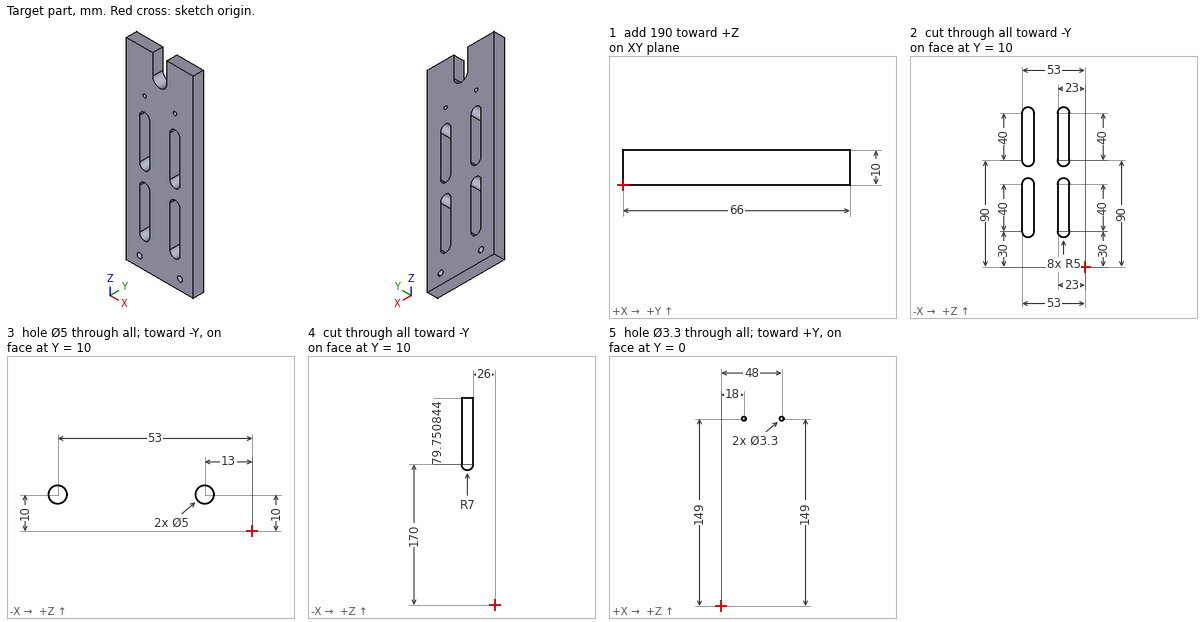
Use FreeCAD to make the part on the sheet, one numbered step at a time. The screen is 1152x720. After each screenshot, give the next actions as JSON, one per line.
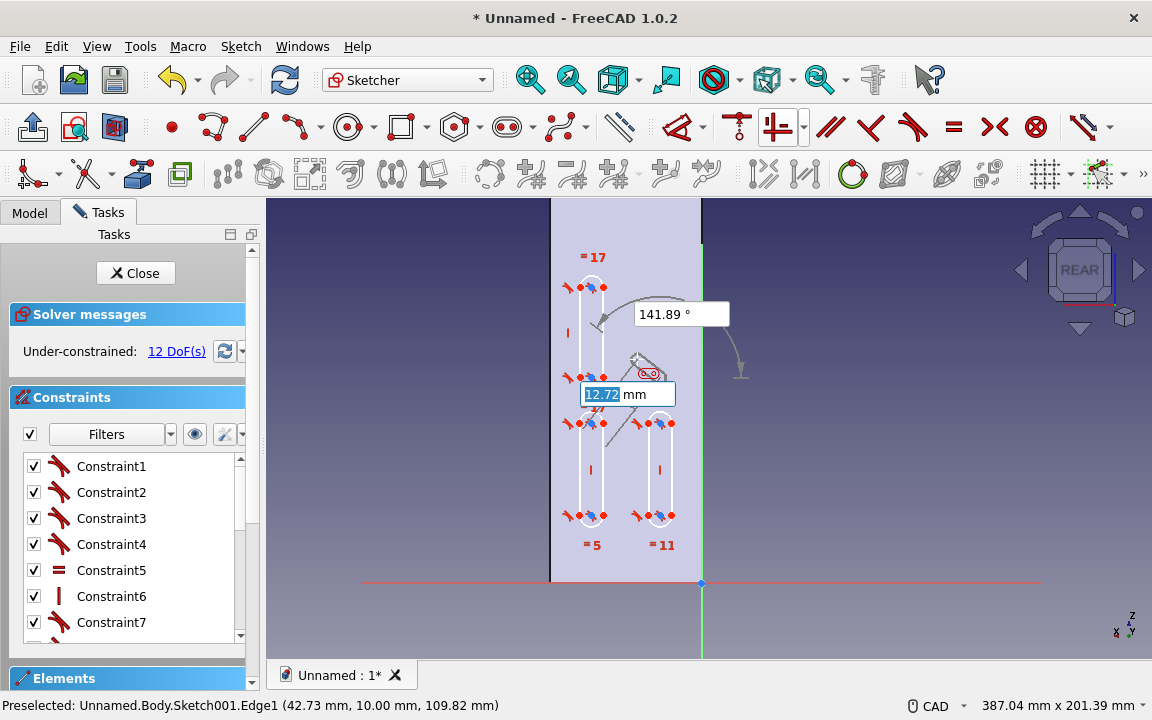
{"action": "left_click", "coordinate": [660, 286]}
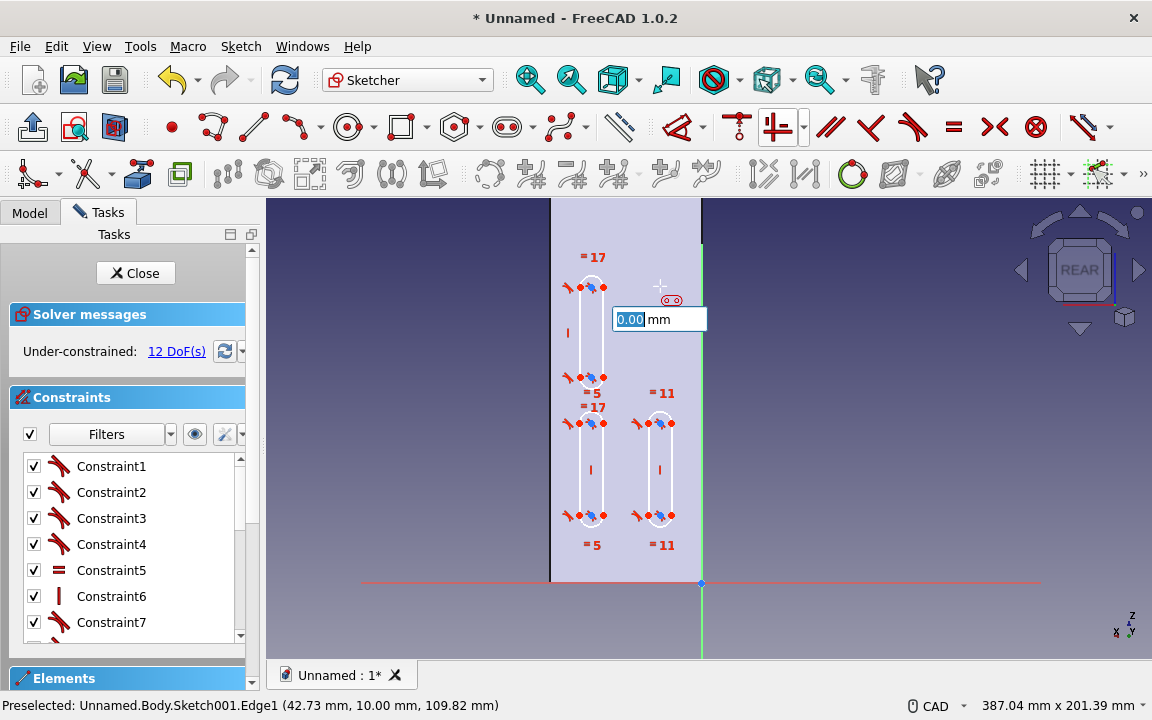
{"action": "scroll", "coordinate": [672, 332], "scroll_direction": "up", "scroll_amount": 2}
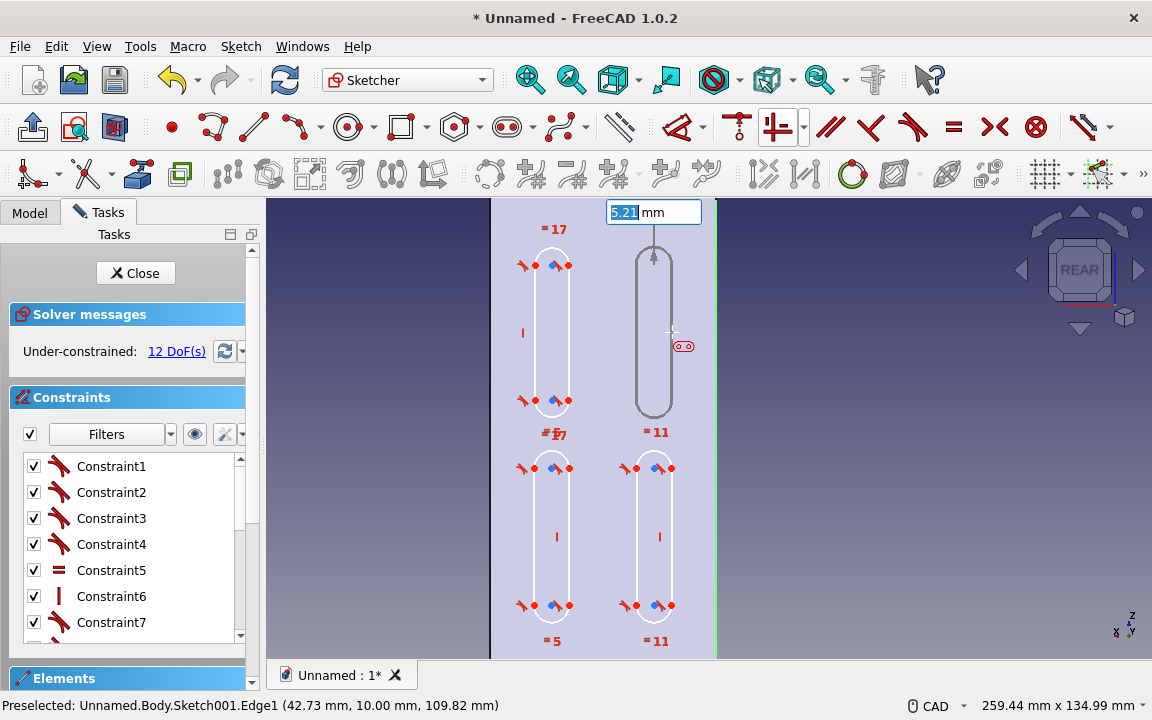
{"action": "left_click", "coordinate": [671, 331]}
{"action": "key", "text": "Escape"}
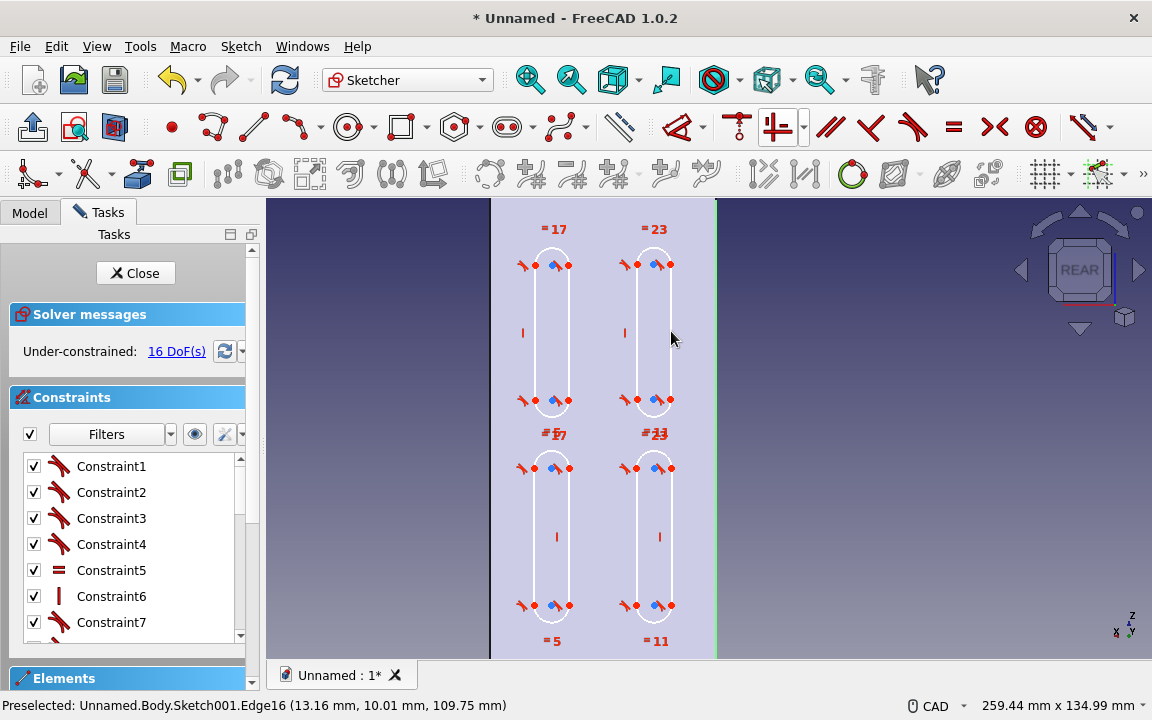
{"action": "left_click", "coordinate": [541, 619]}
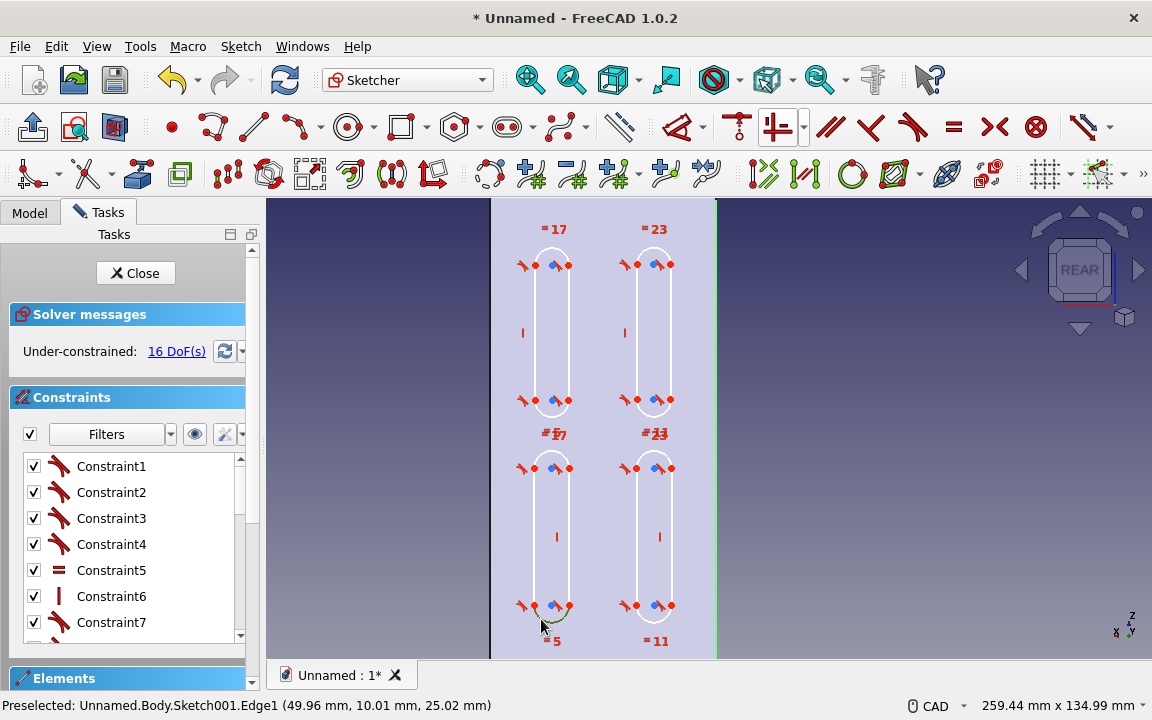
{"action": "left_click", "coordinate": [644, 619]}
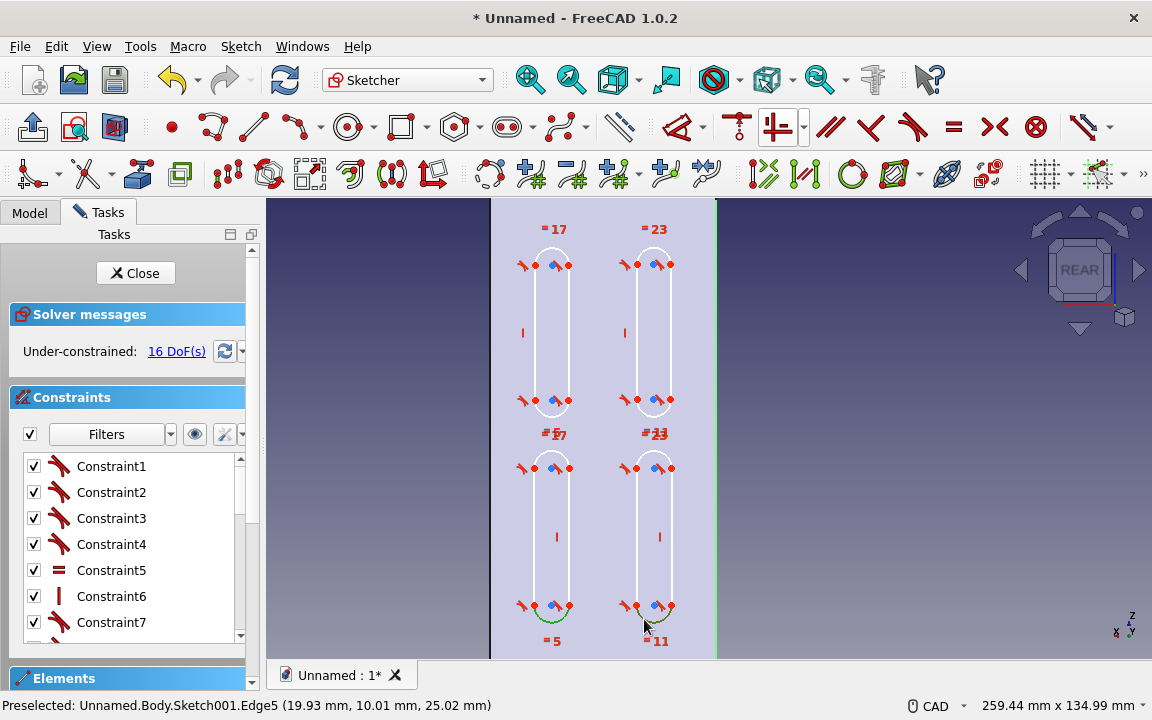
{"action": "left_click", "coordinate": [542, 414]}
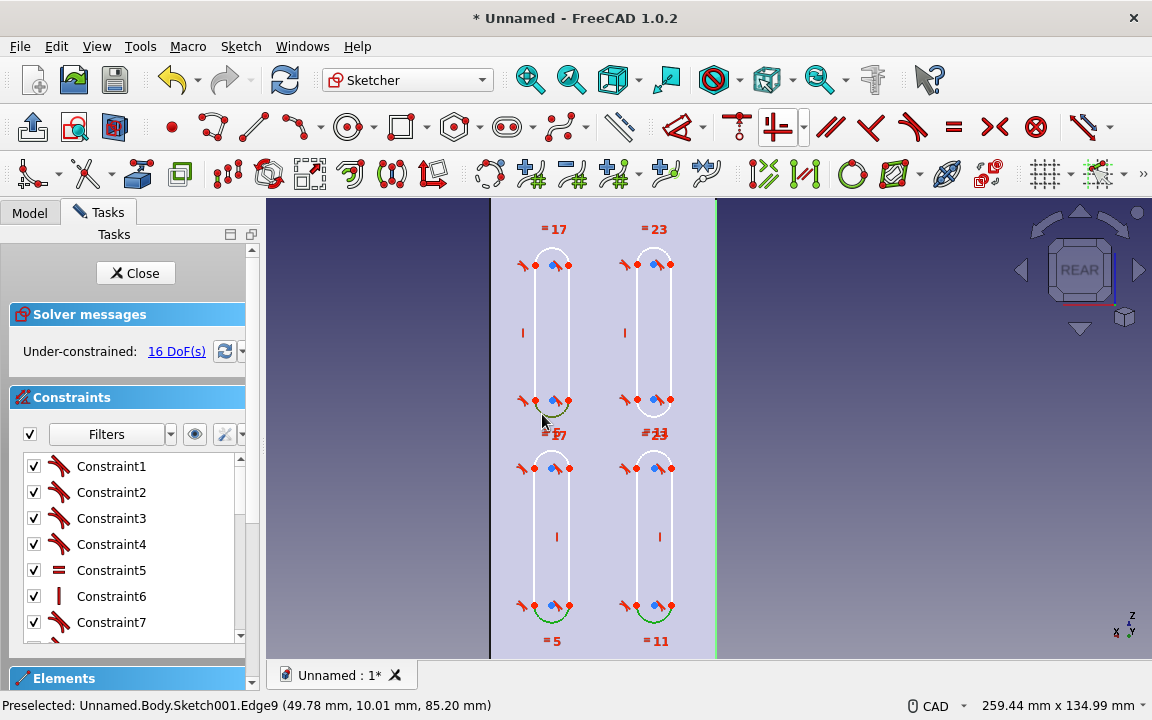
{"action": "left_click", "coordinate": [644, 414]}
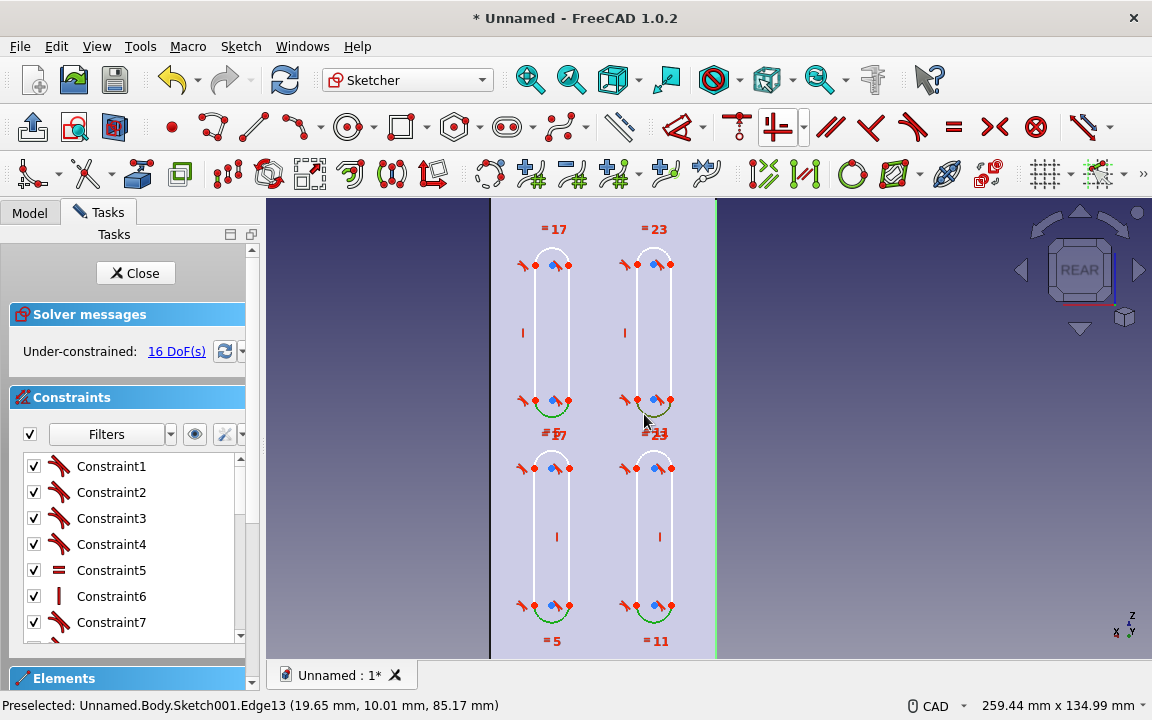
{"action": "left_click", "coordinate": [954, 128]}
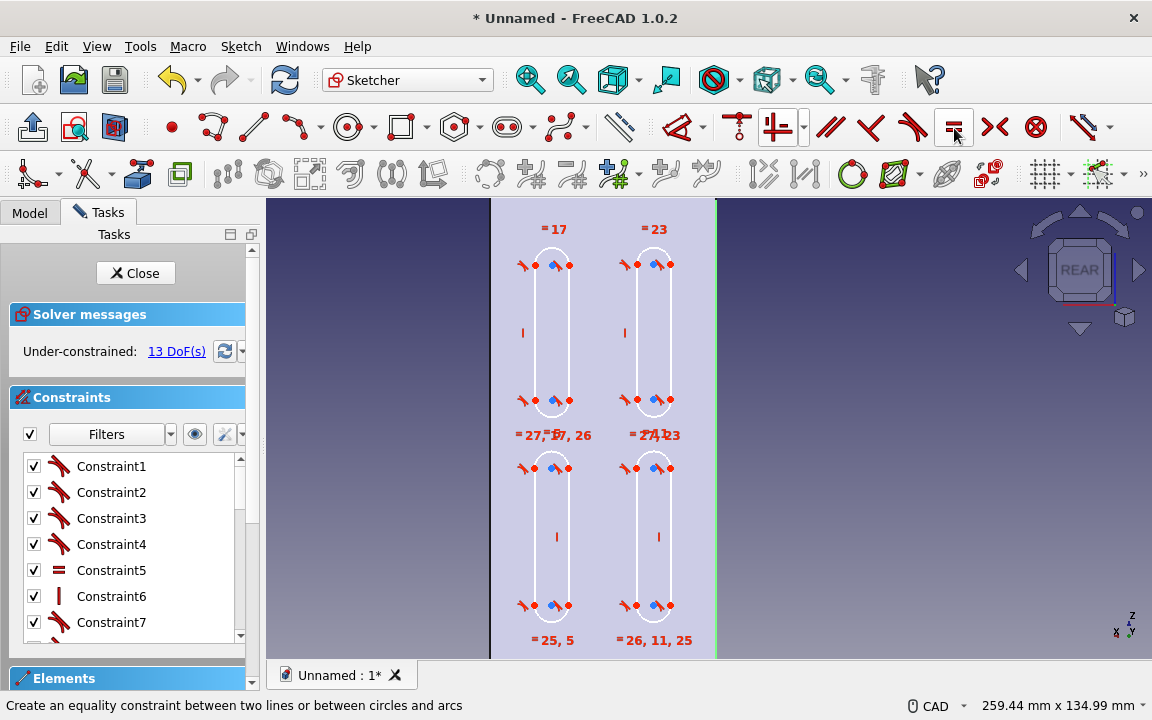
{"action": "left_click", "coordinate": [676, 128]}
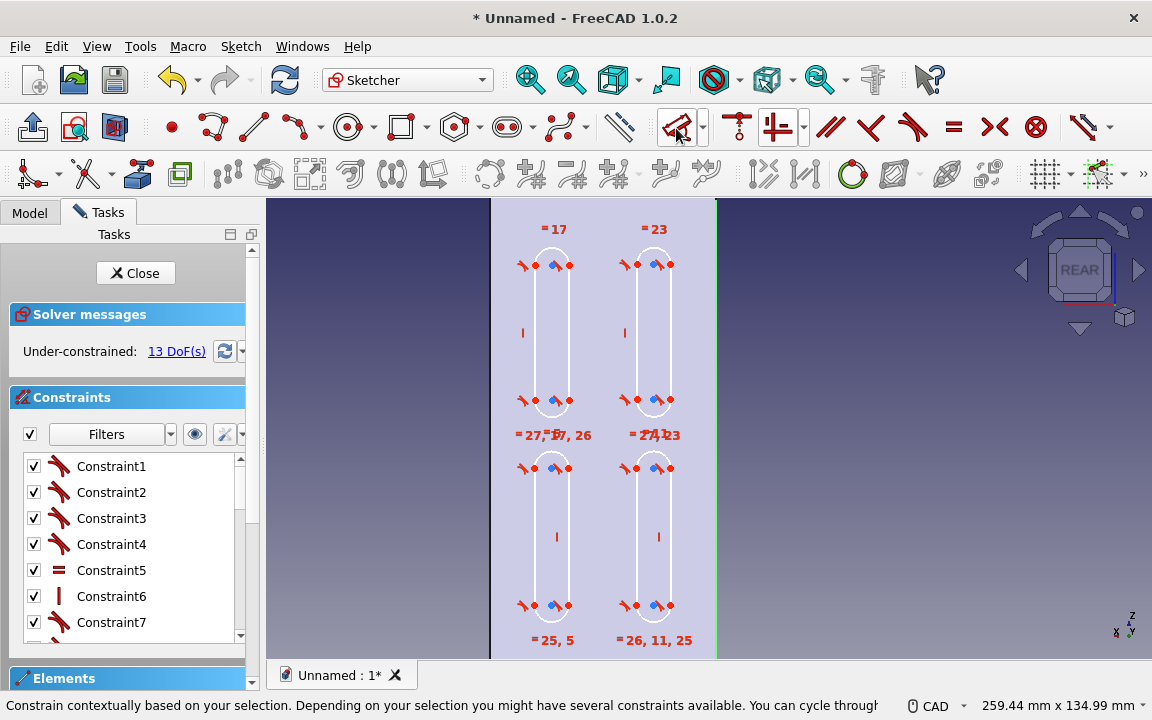
{"action": "scroll", "coordinate": [542, 619], "scroll_direction": "up", "scroll_amount": 5}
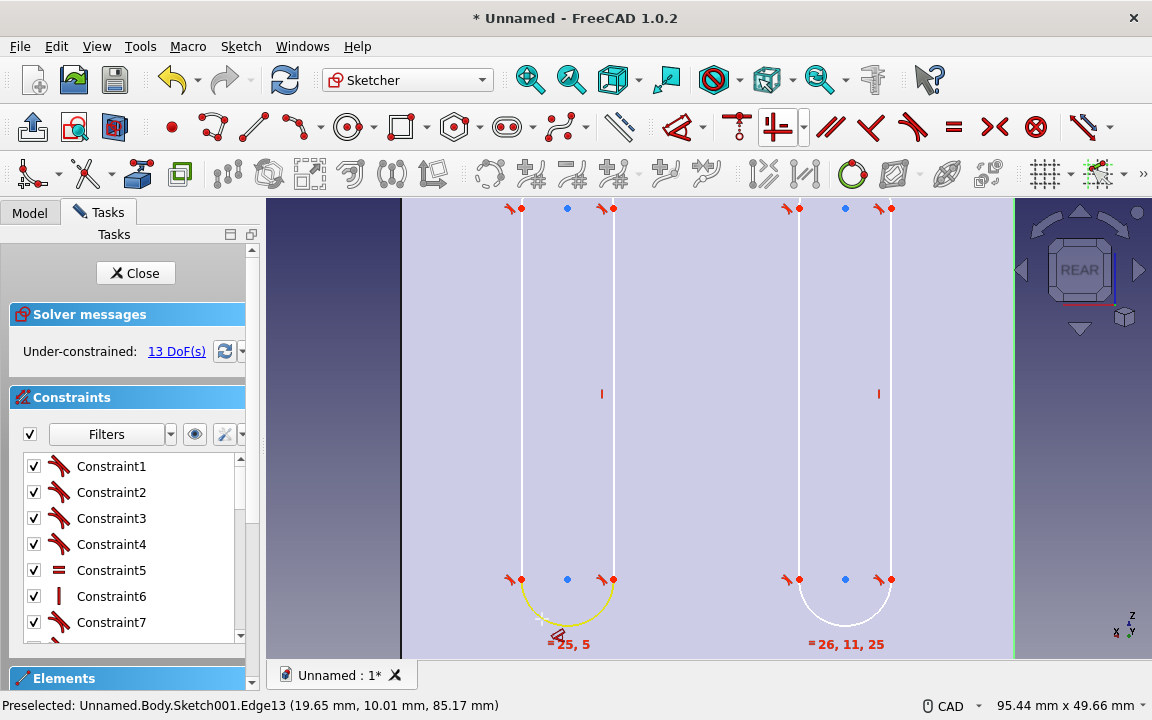
{"action": "left_click", "coordinate": [541, 617]}
{"action": "left_click", "coordinate": [498, 614]}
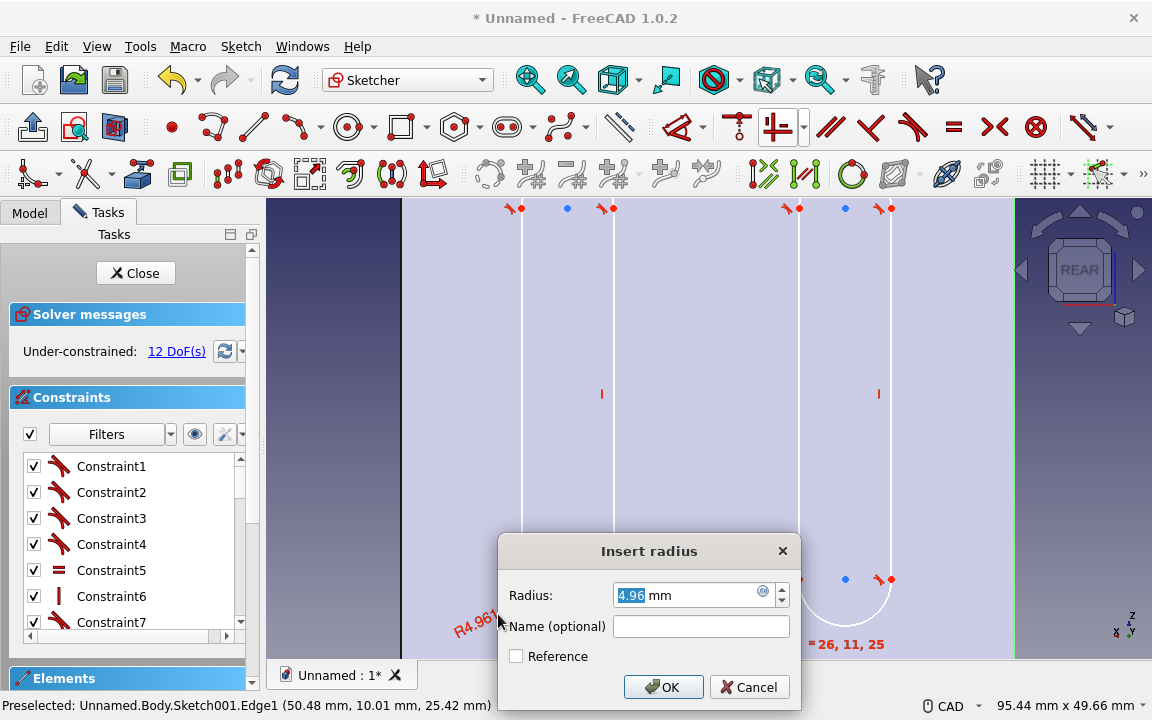
{"action": "type", "text": "5"}
{"action": "key", "text": "Return"}